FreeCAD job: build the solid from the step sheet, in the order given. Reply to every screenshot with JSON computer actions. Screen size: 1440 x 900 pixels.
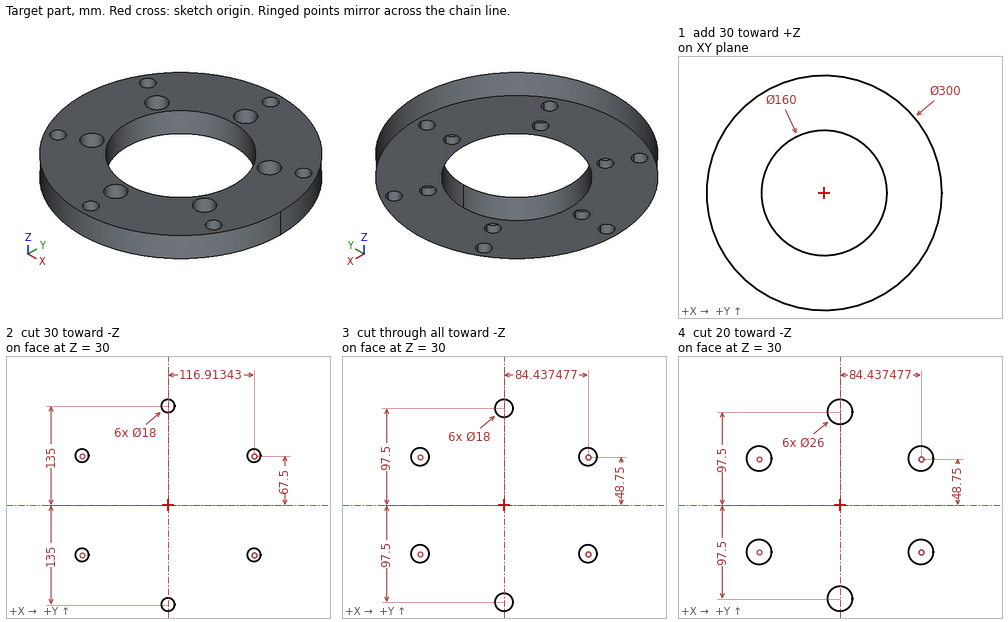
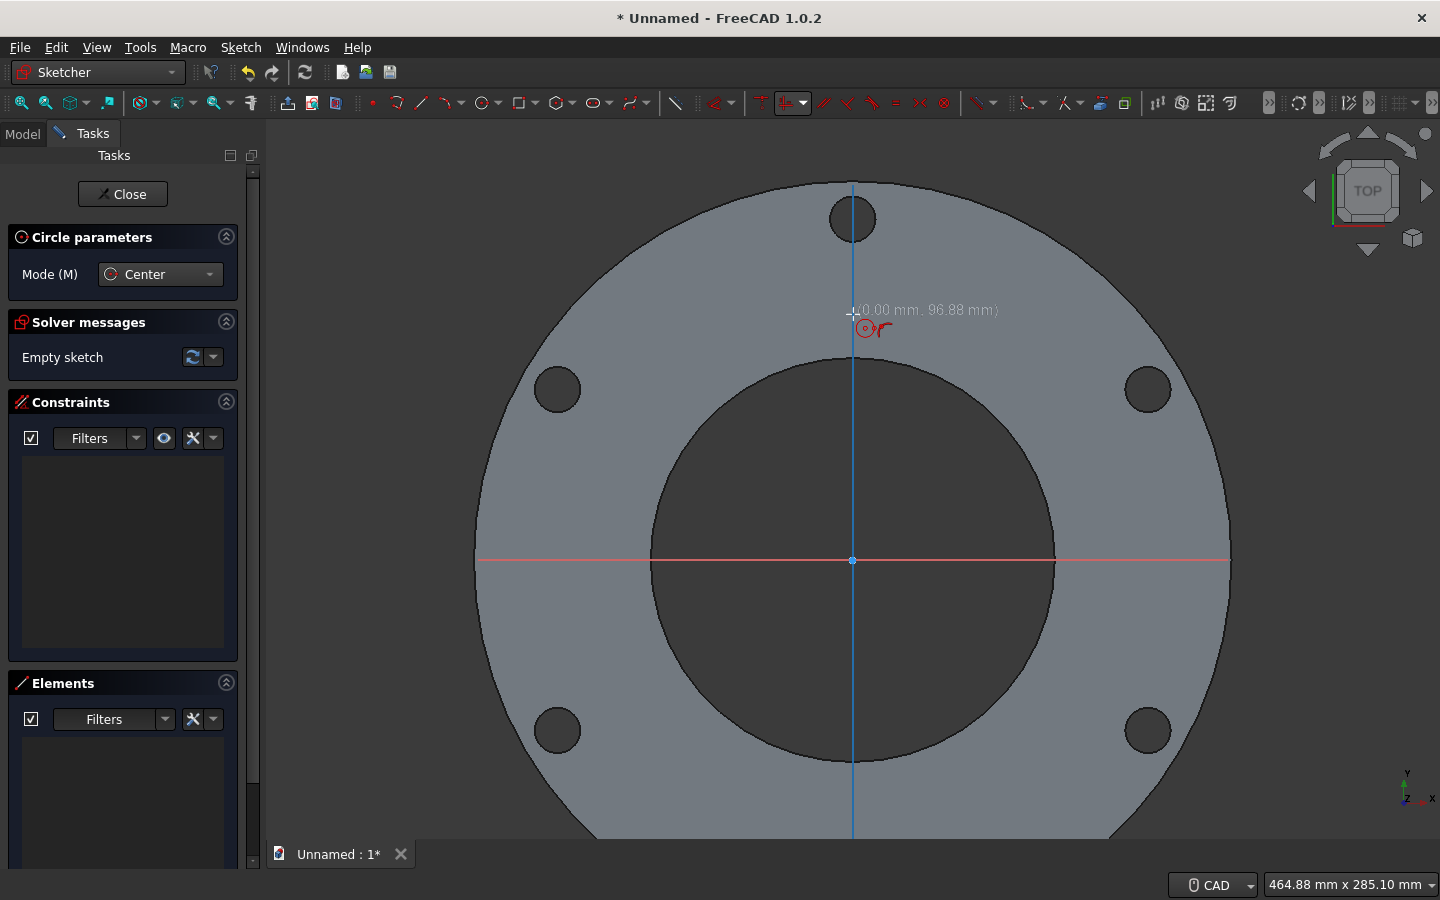
{"action": "left_click", "coordinate": [853, 314]}
{"action": "left_click", "coordinate": [869, 298]}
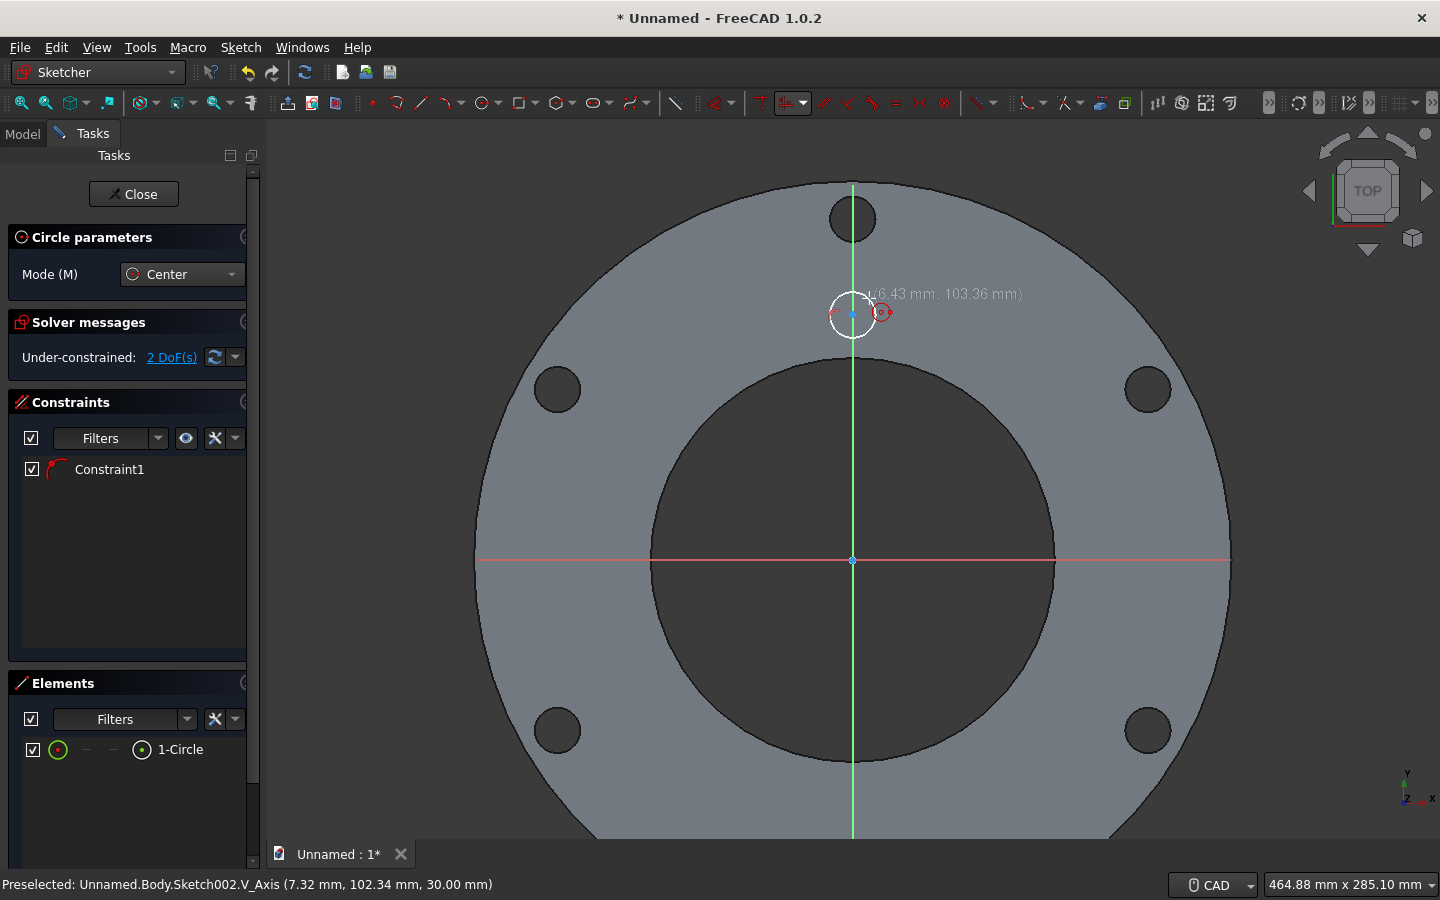
{"action": "left_click", "coordinate": [1066, 437]}
{"action": "left_click", "coordinate": [1082, 421]}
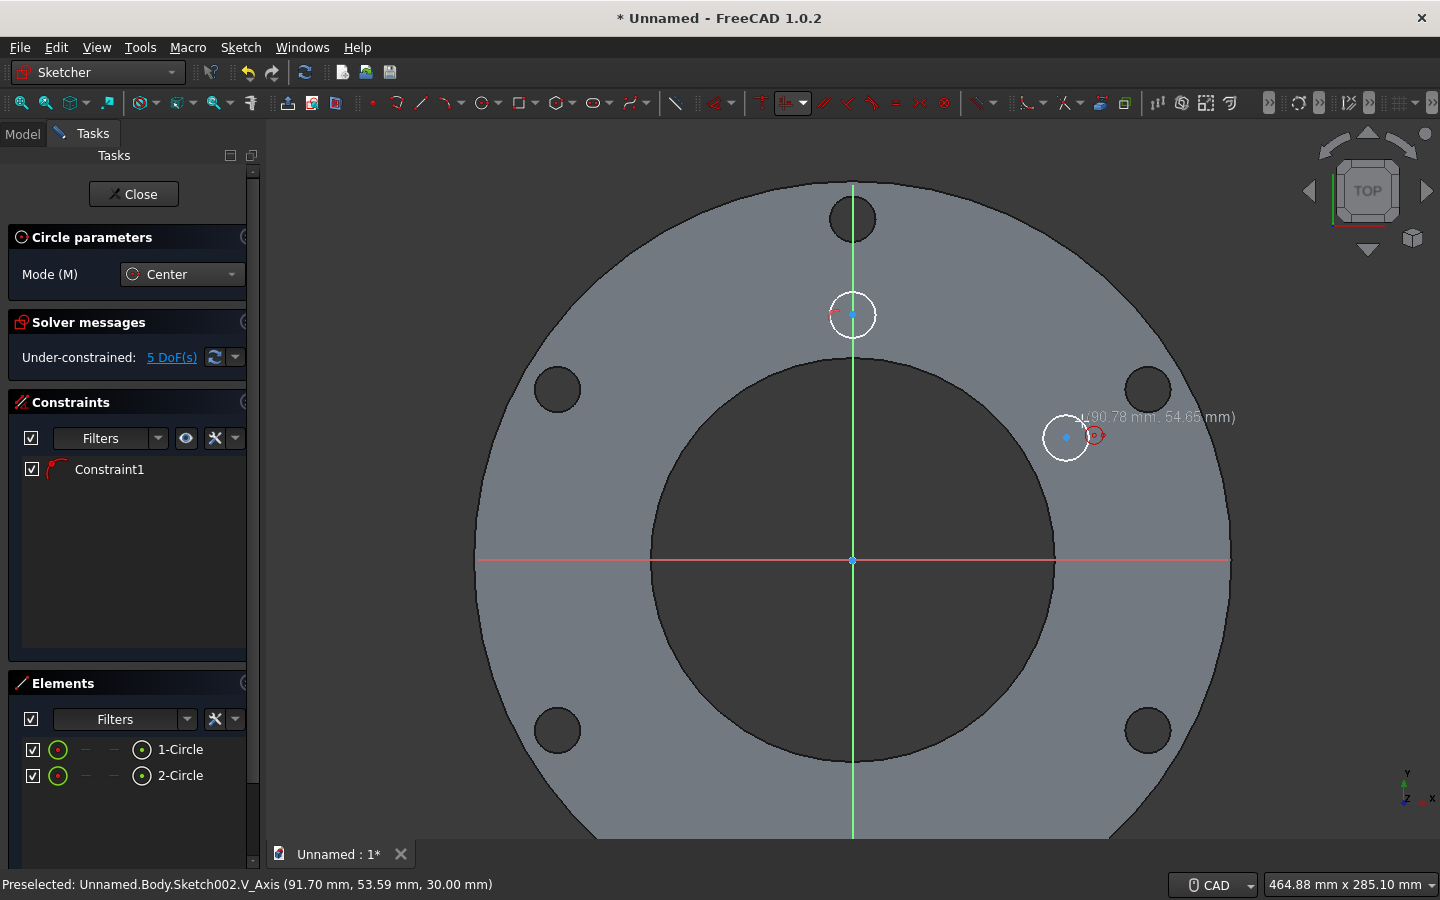
{"action": "left_click", "coordinate": [1066, 683]}
{"action": "left_click", "coordinate": [1082, 667]}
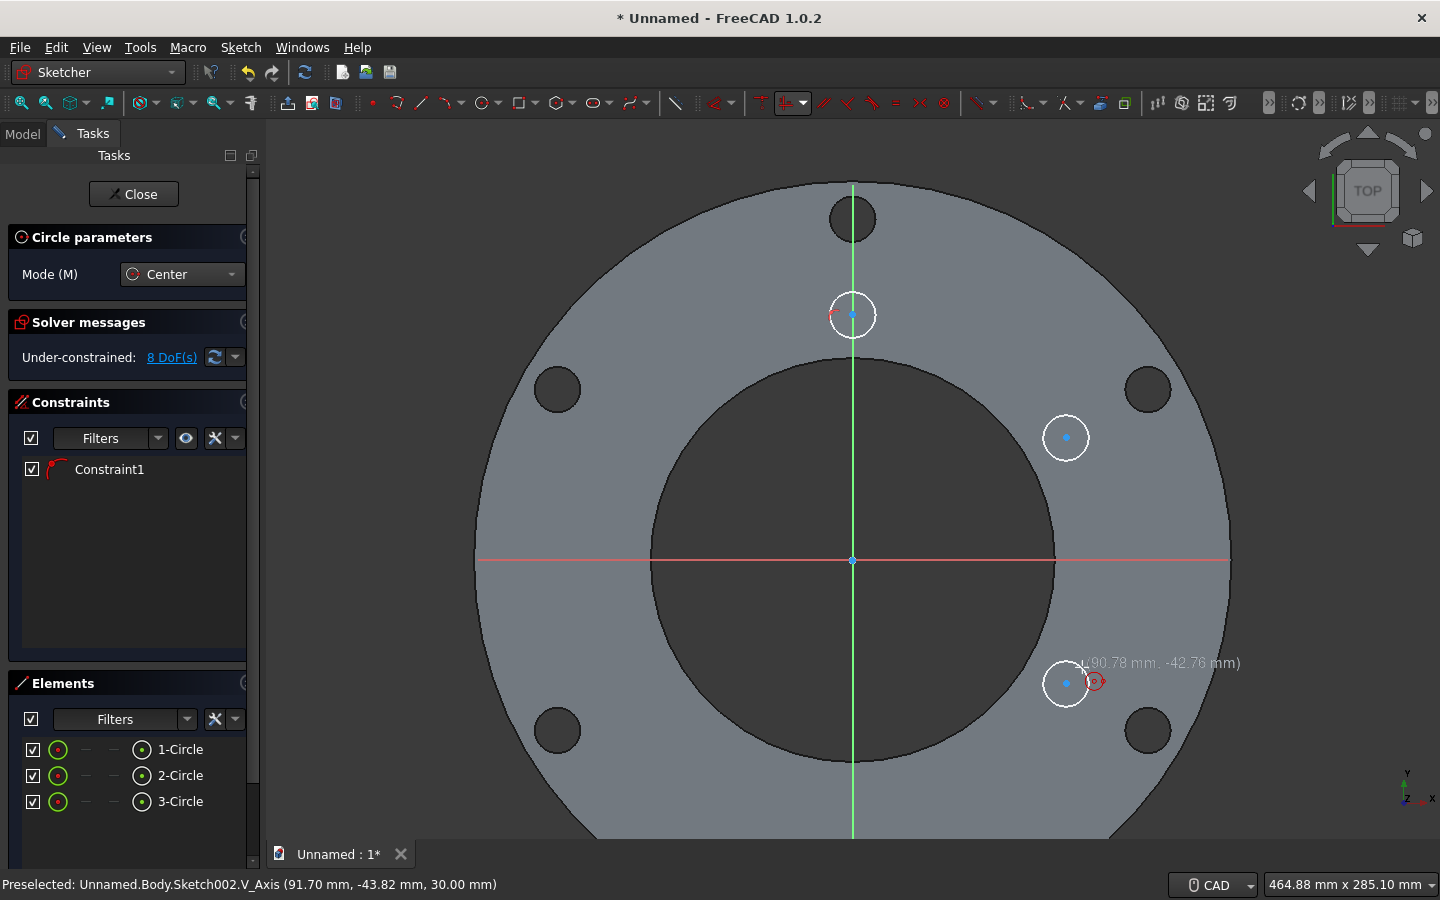
{"action": "left_click", "coordinate": [853, 806]}
{"action": "left_click", "coordinate": [869, 790]}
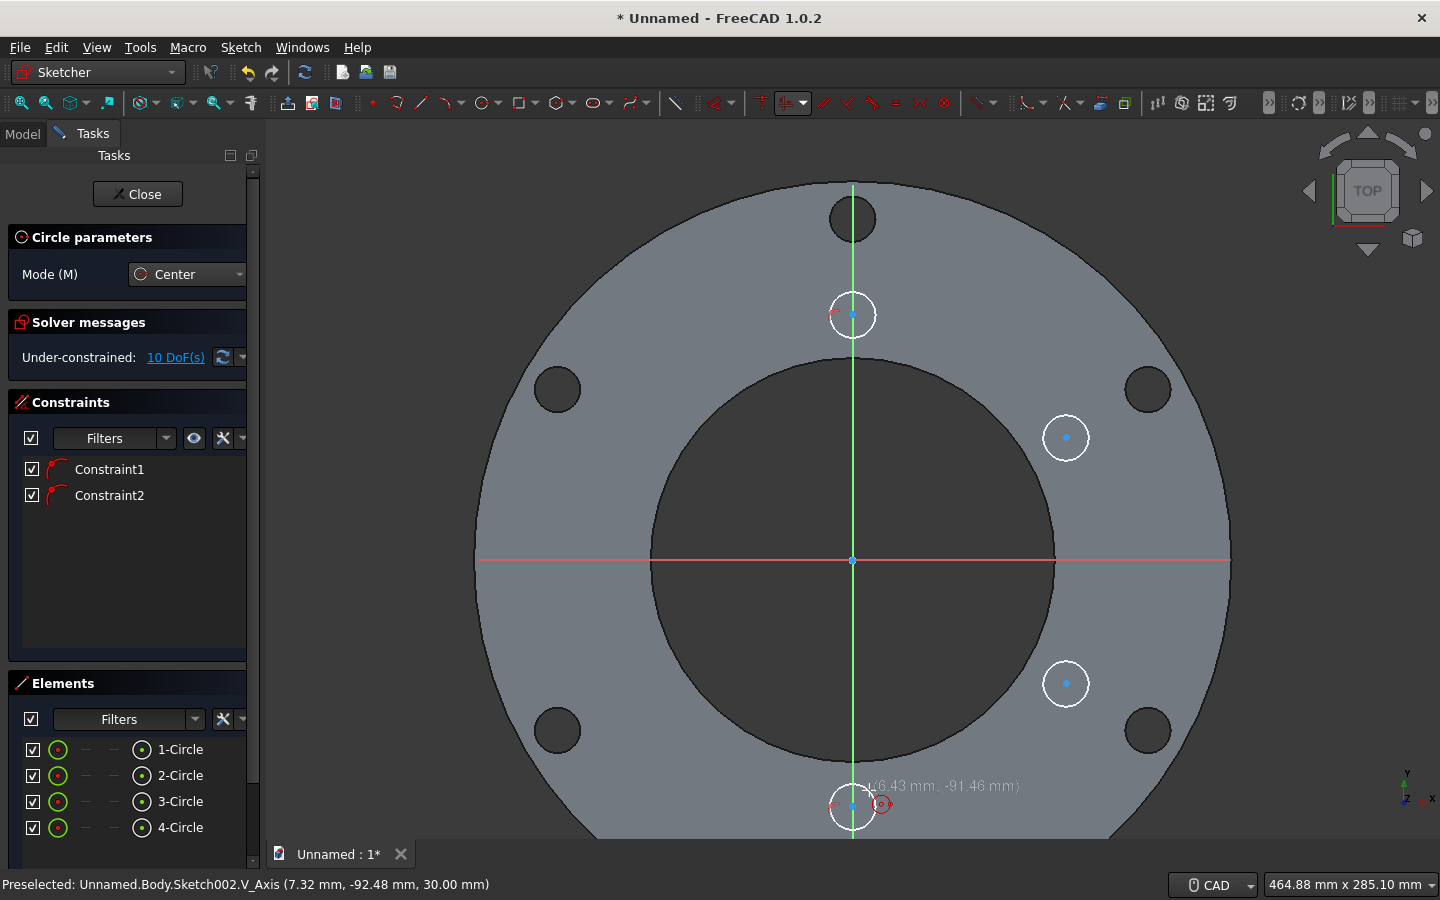
{"action": "left_click", "coordinate": [640, 683]}
{"action": "left_click", "coordinate": [656, 667]}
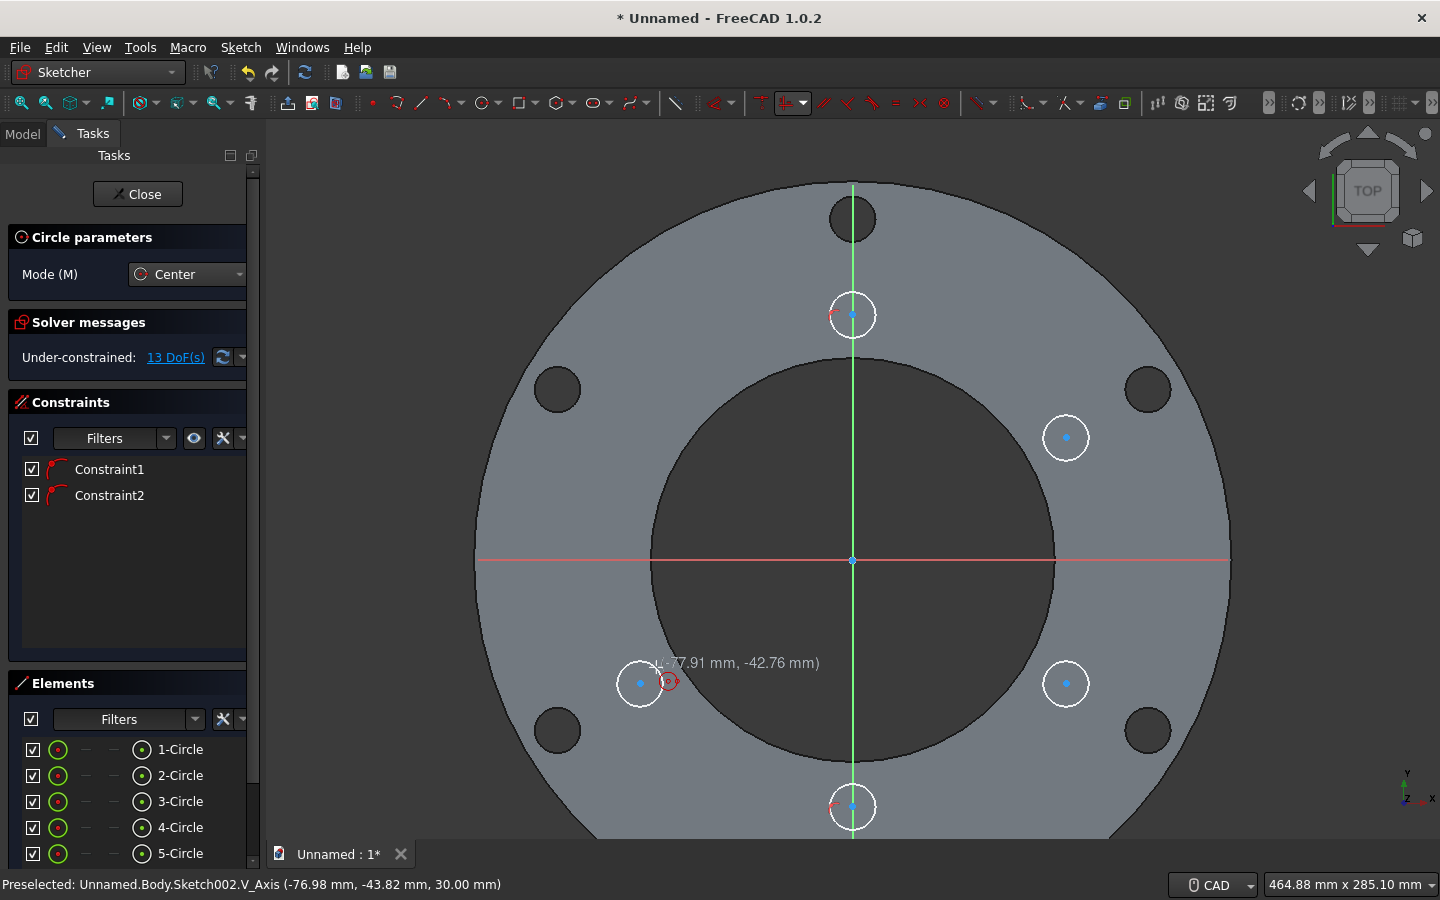
{"action": "left_click", "coordinate": [640, 437]}
{"action": "left_click", "coordinate": [656, 421]}
{"action": "key", "text": "Escape"}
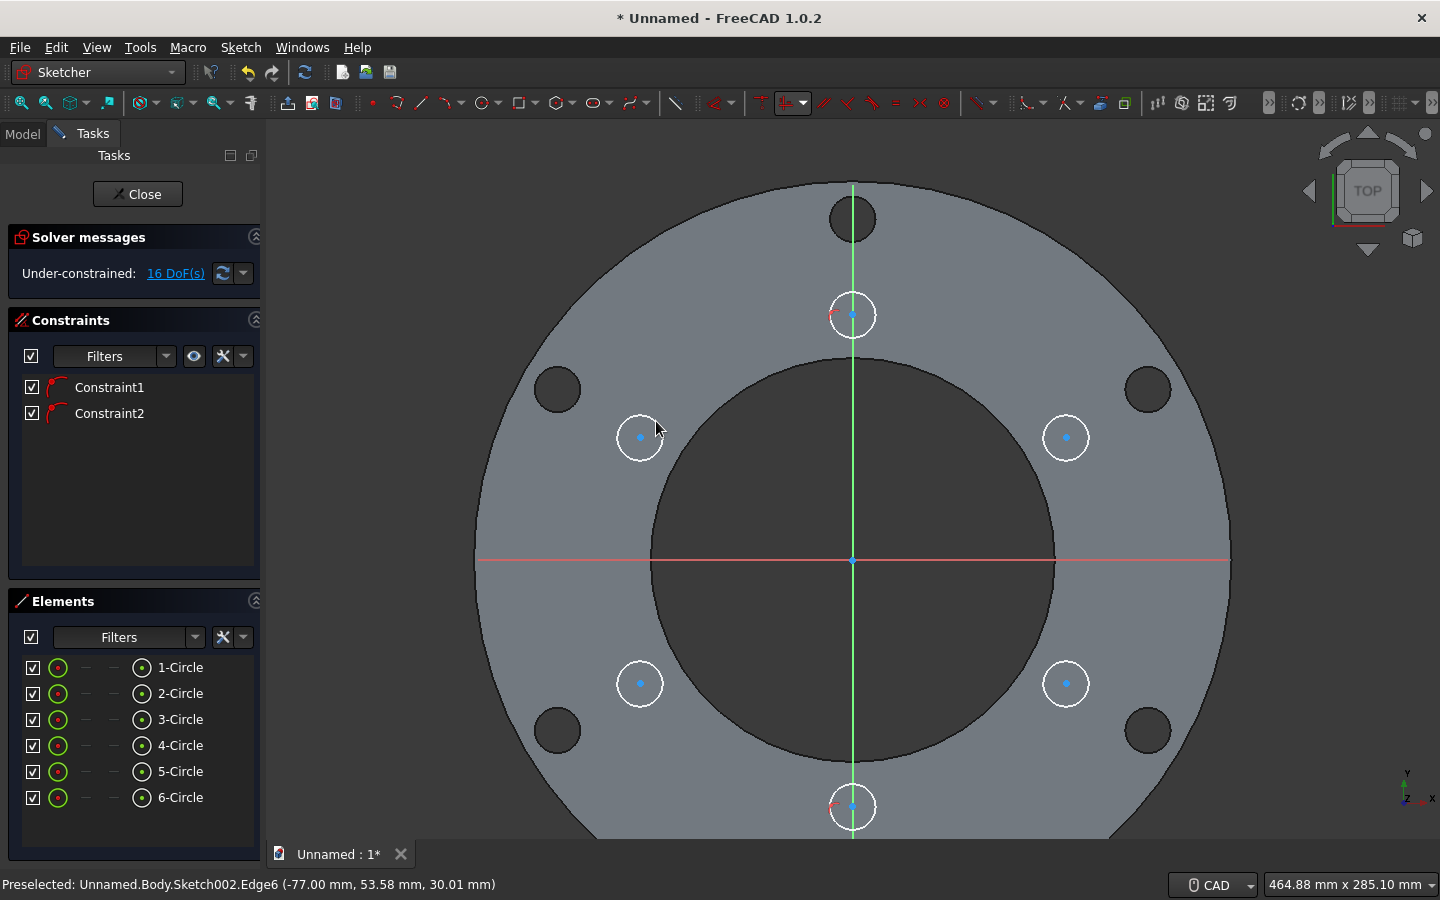
{"action": "left_click", "coordinate": [869, 299]}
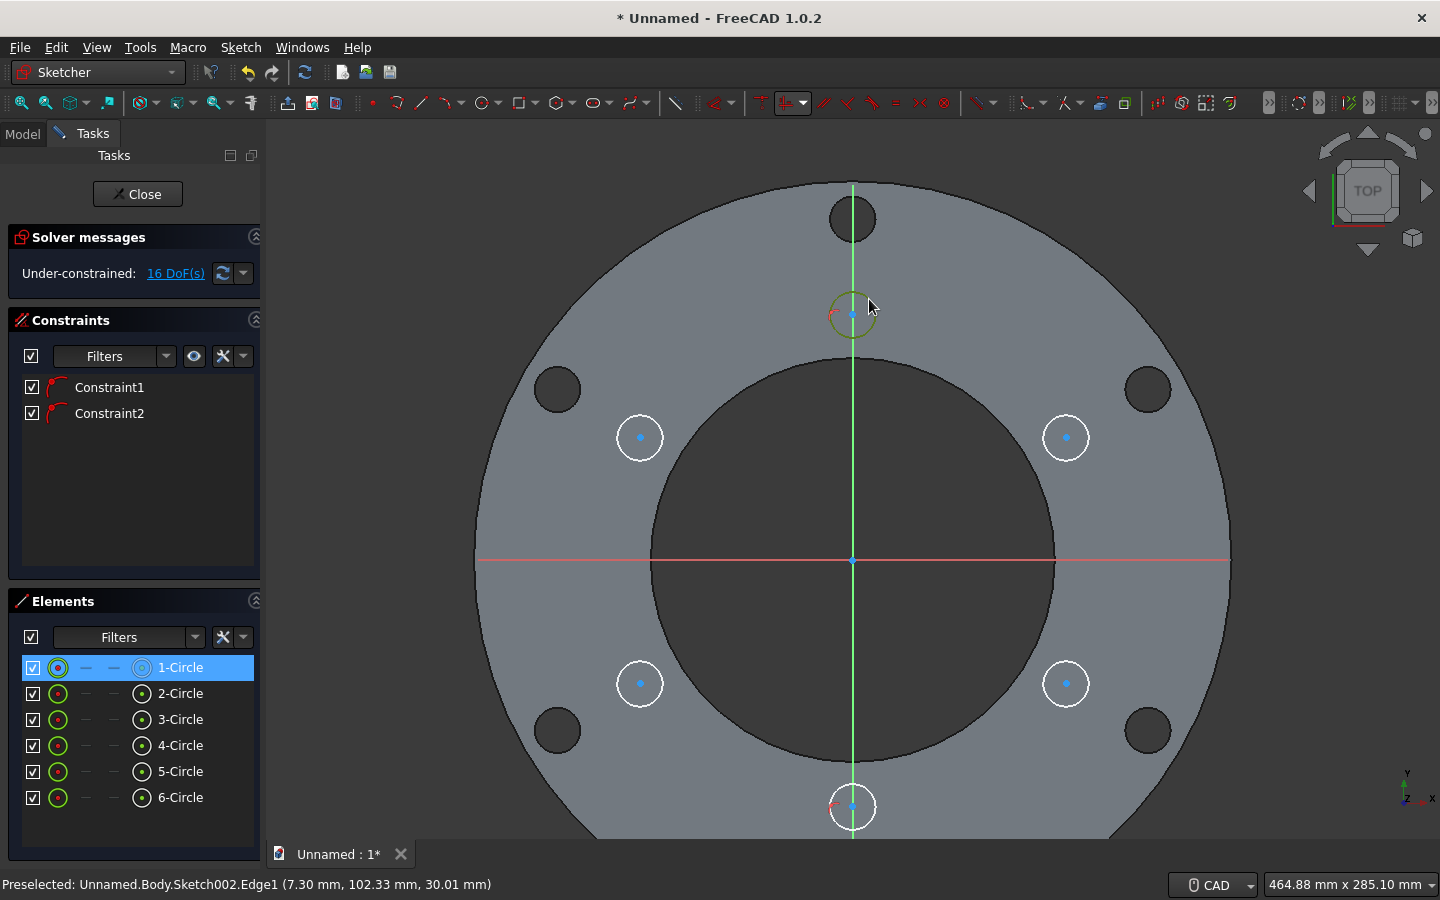
{"action": "left_click", "coordinate": [1082, 422]}